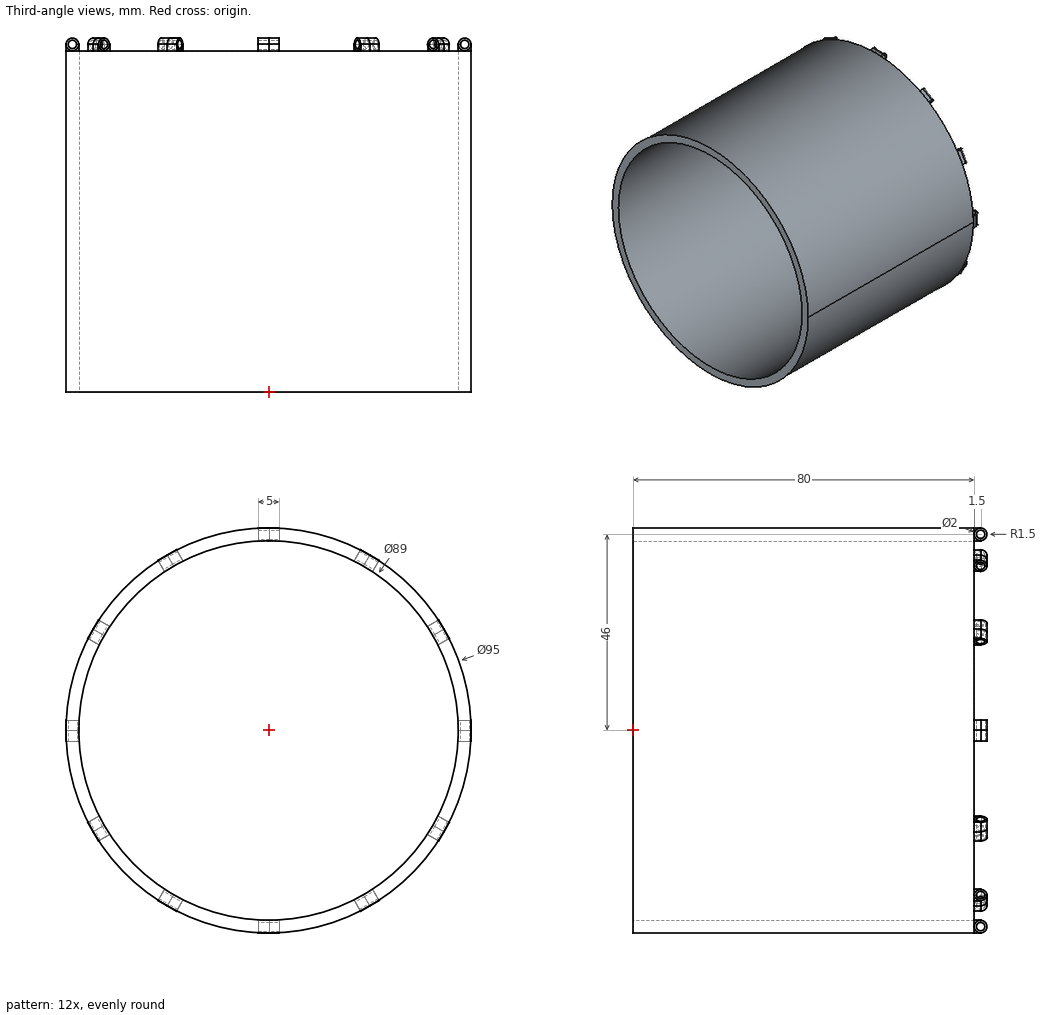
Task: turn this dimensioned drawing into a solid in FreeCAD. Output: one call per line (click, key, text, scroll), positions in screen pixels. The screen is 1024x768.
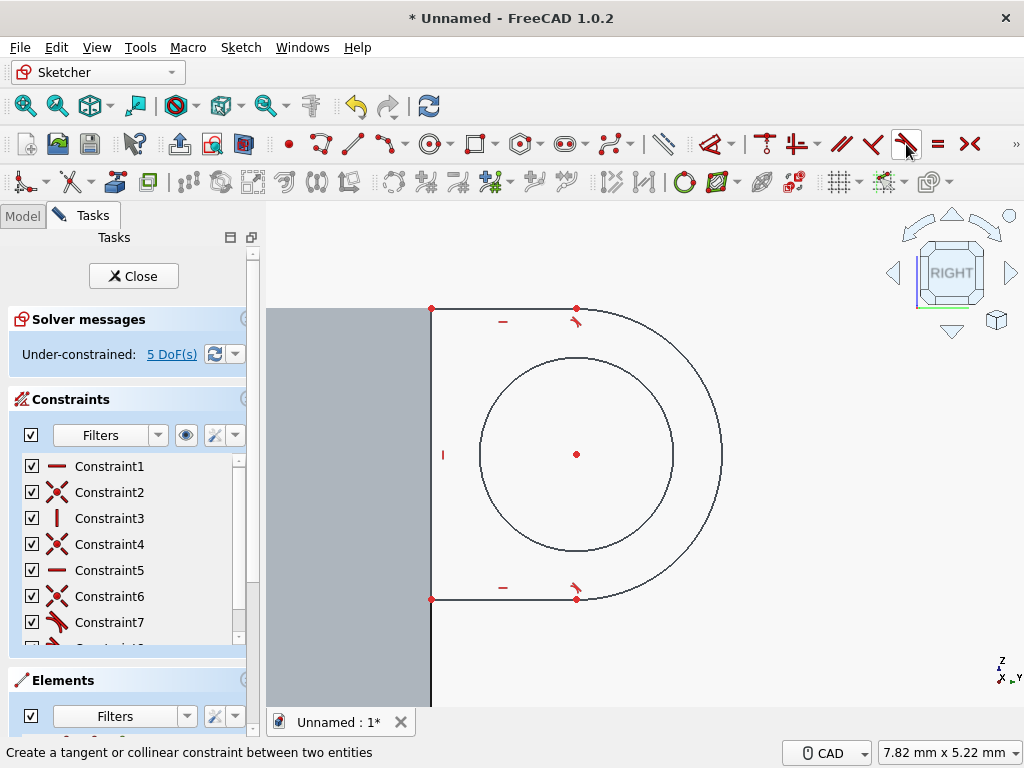
click(710, 144)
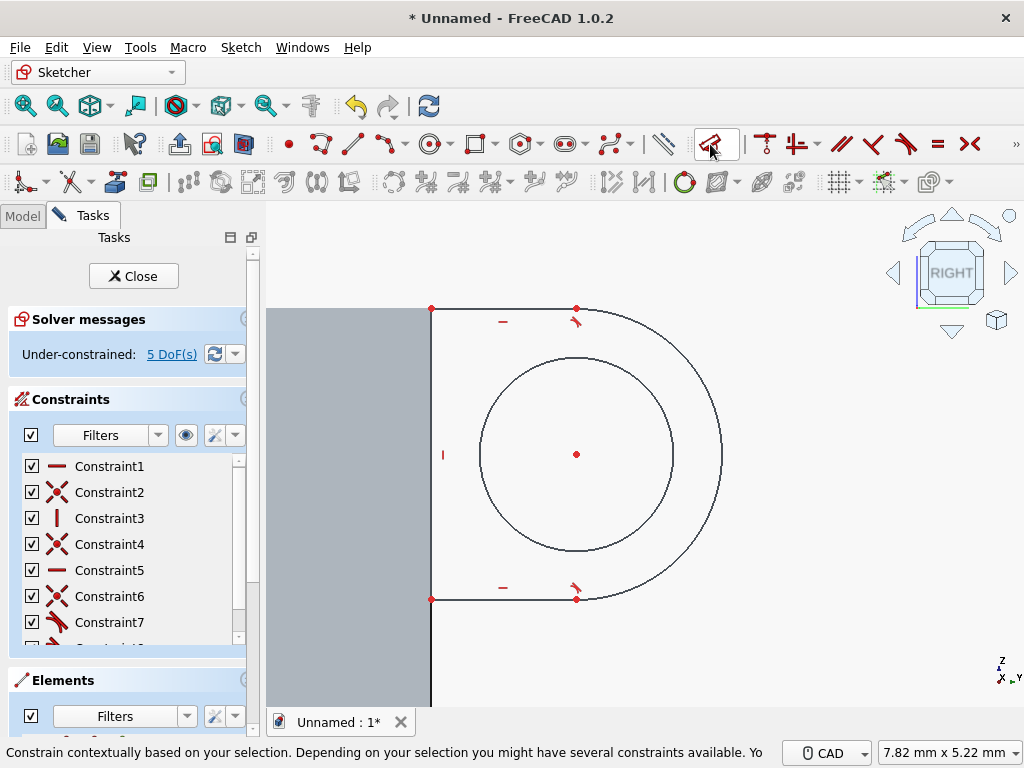
click(694, 540)
click(720, 559)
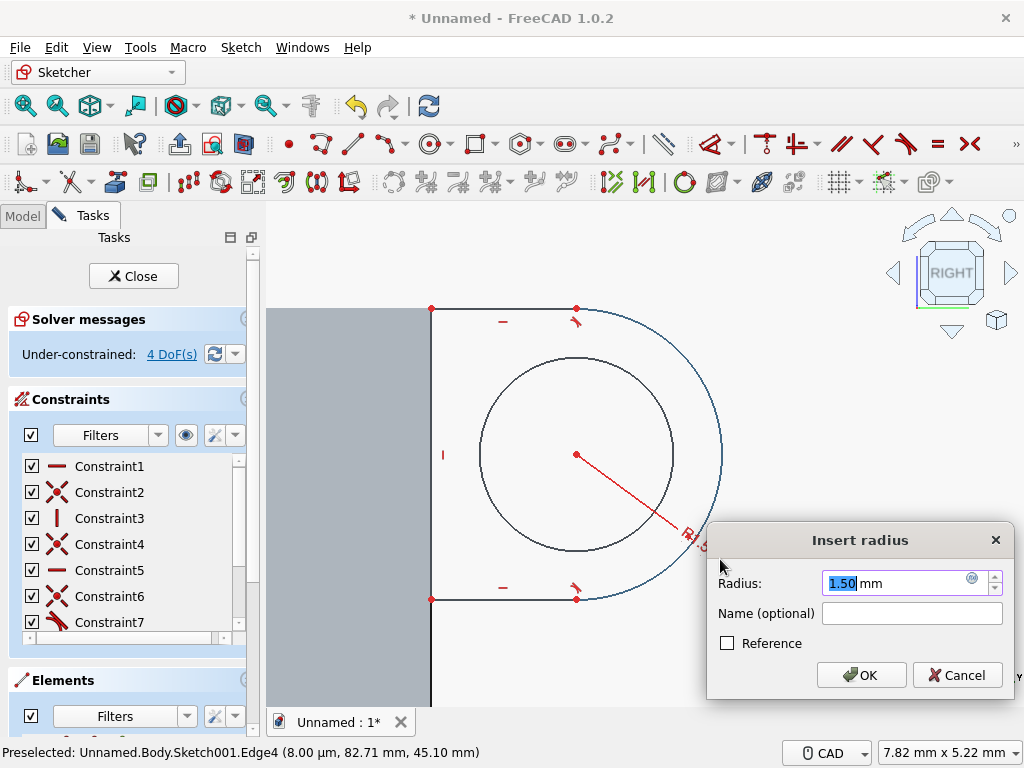
text(1.5)
key(Return)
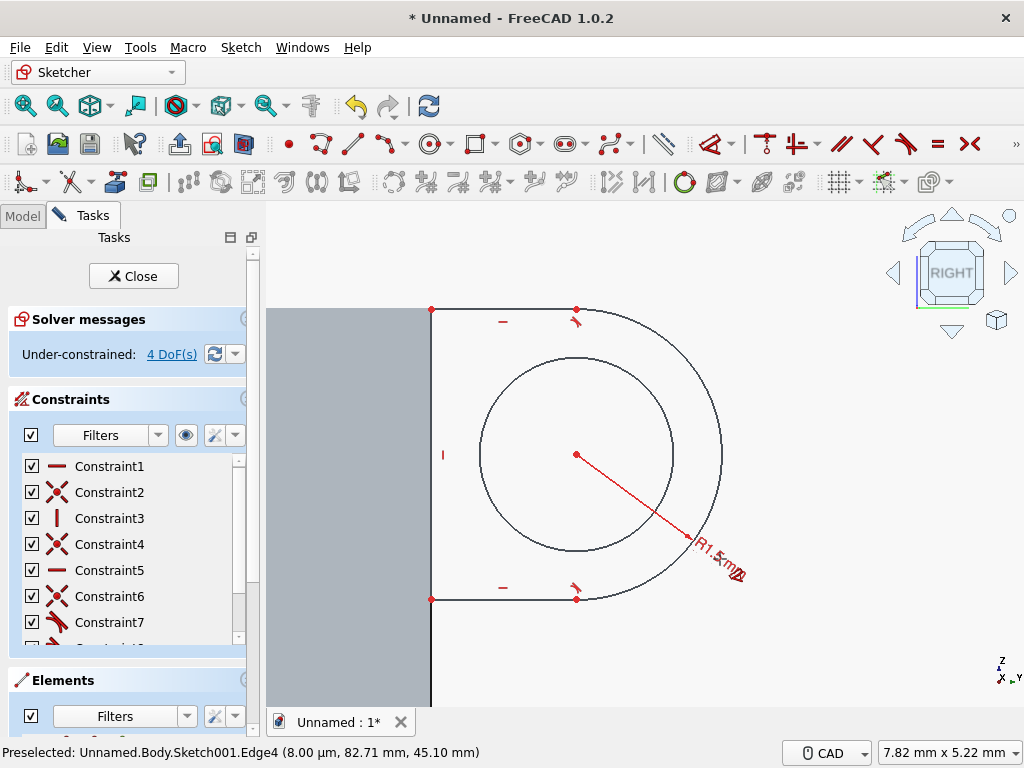
click(645, 386)
click(668, 363)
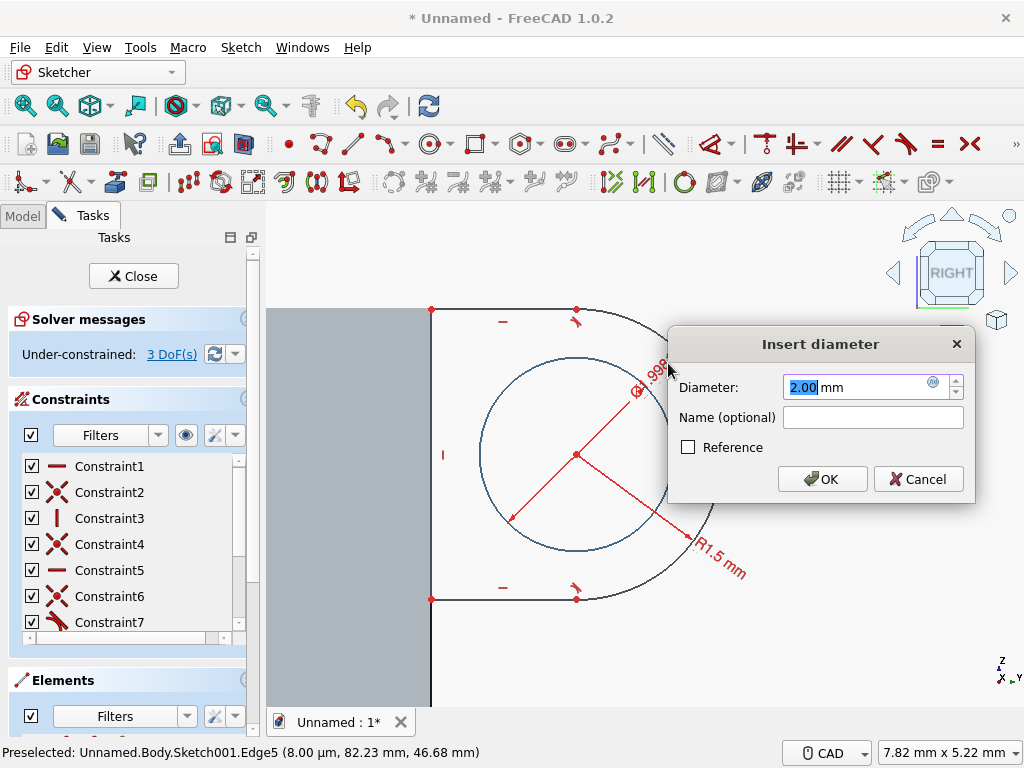
text(2)
key(Return)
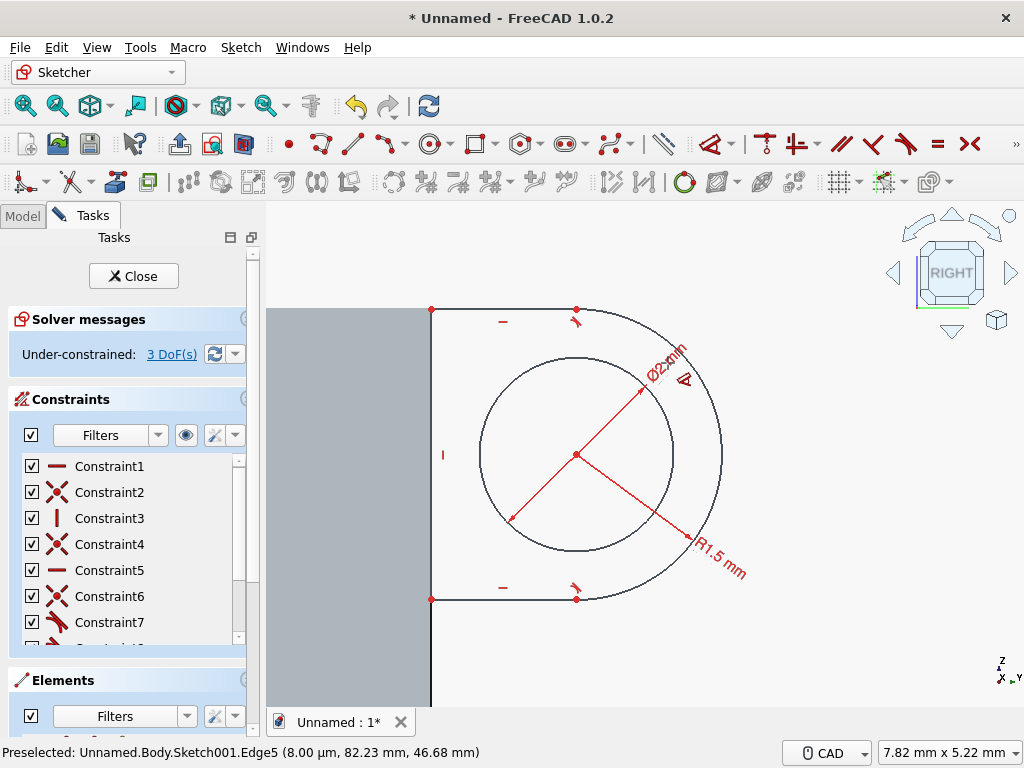
click(576, 455)
click(610, 567)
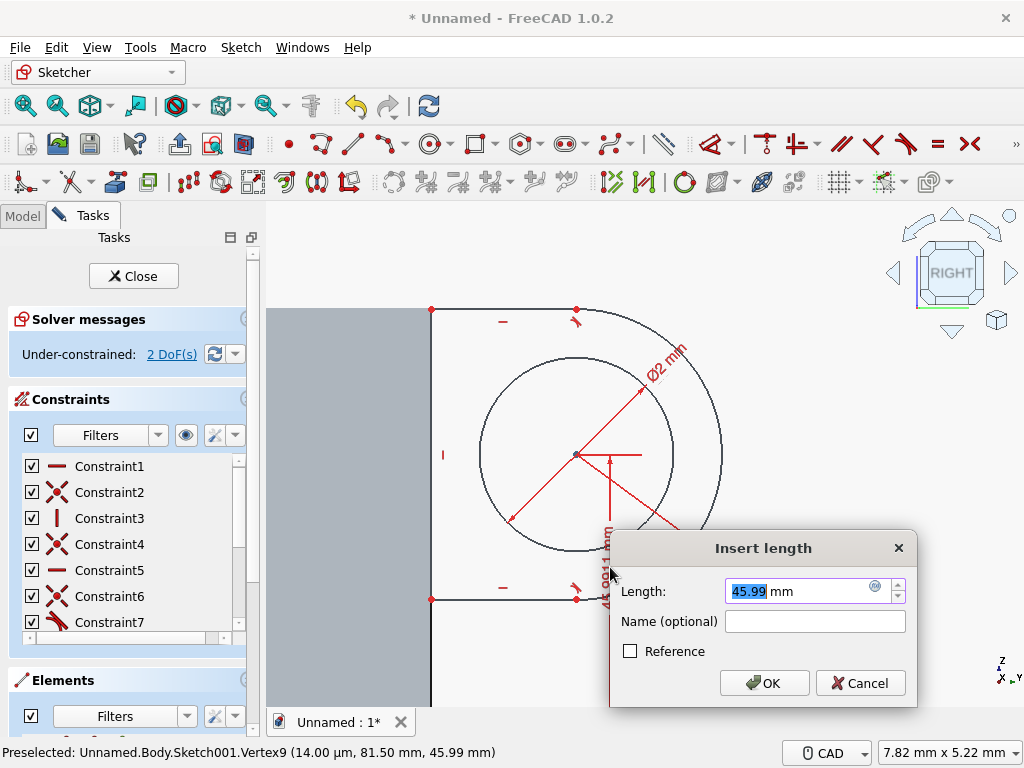
text(46)
key(Return)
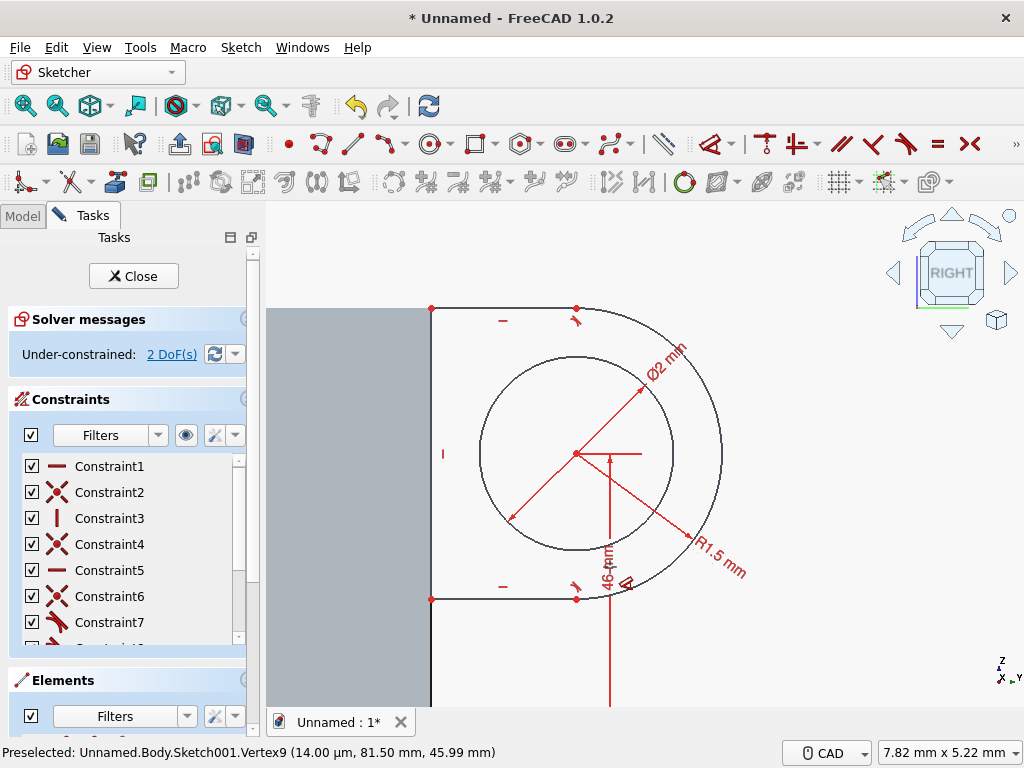
click(533, 308)
click(504, 274)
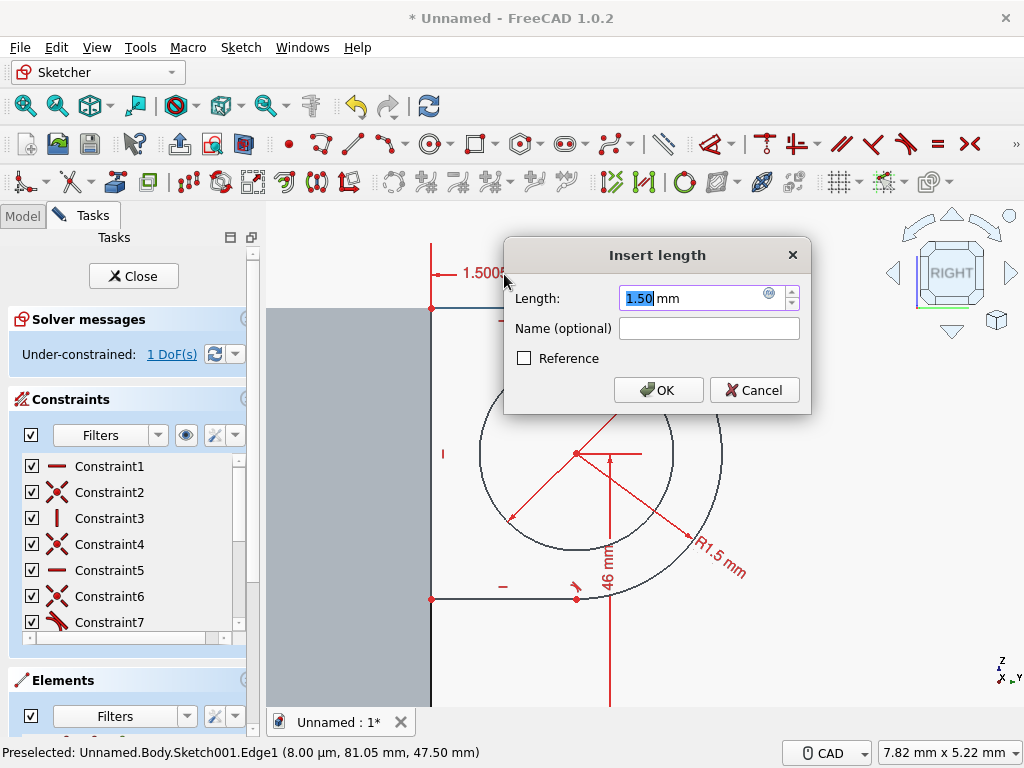
text(1.5)
key(Return)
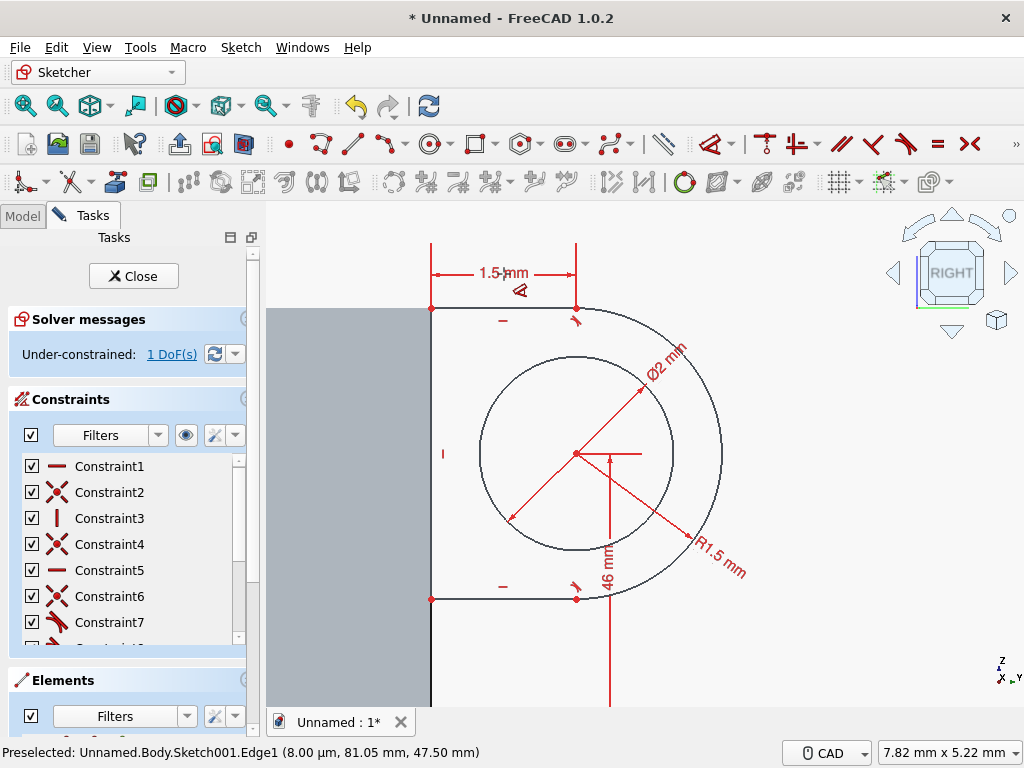
click(431, 308)
click(363, 274)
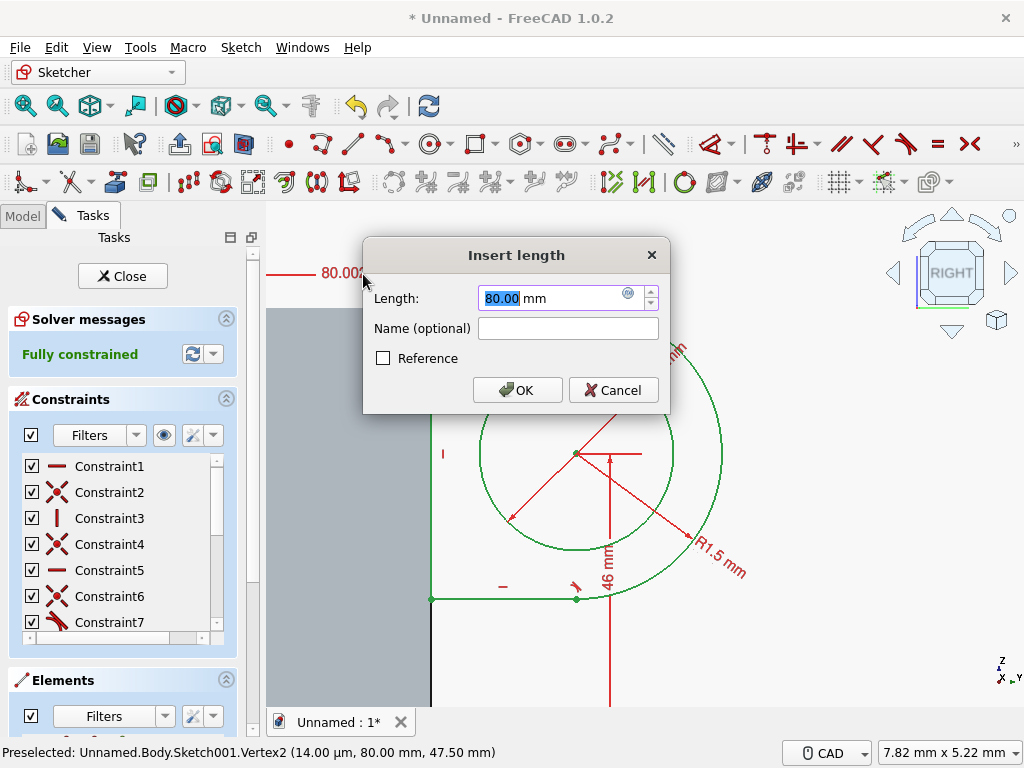
text(80)
key(Return)
key(Escape)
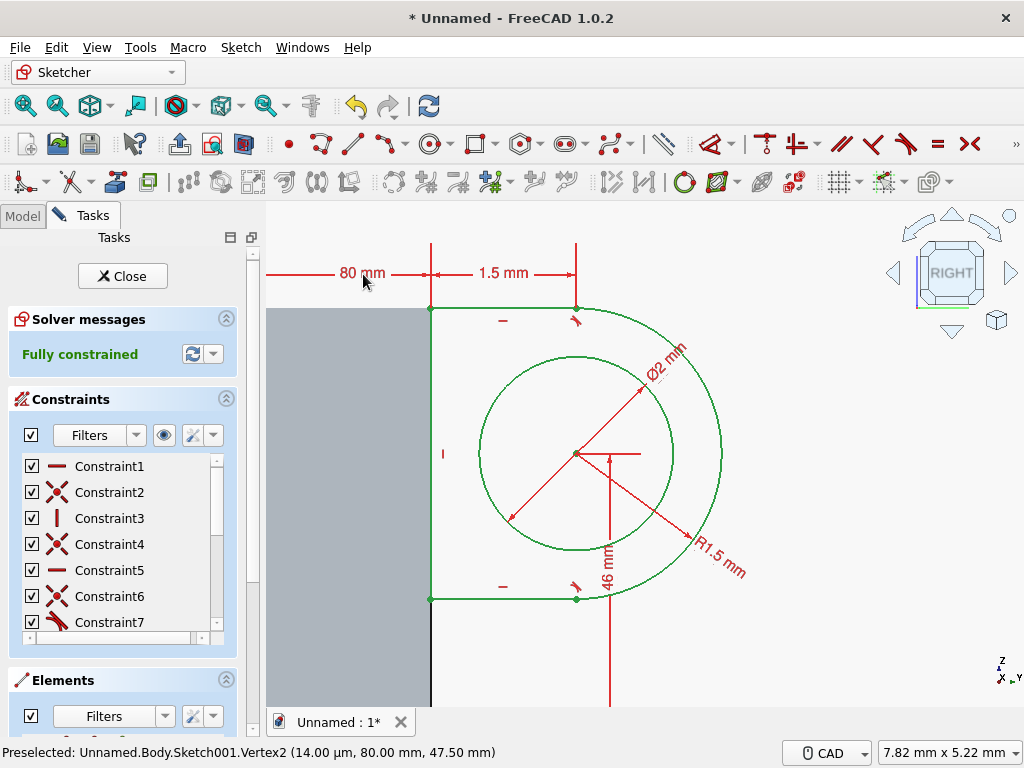
click(123, 276)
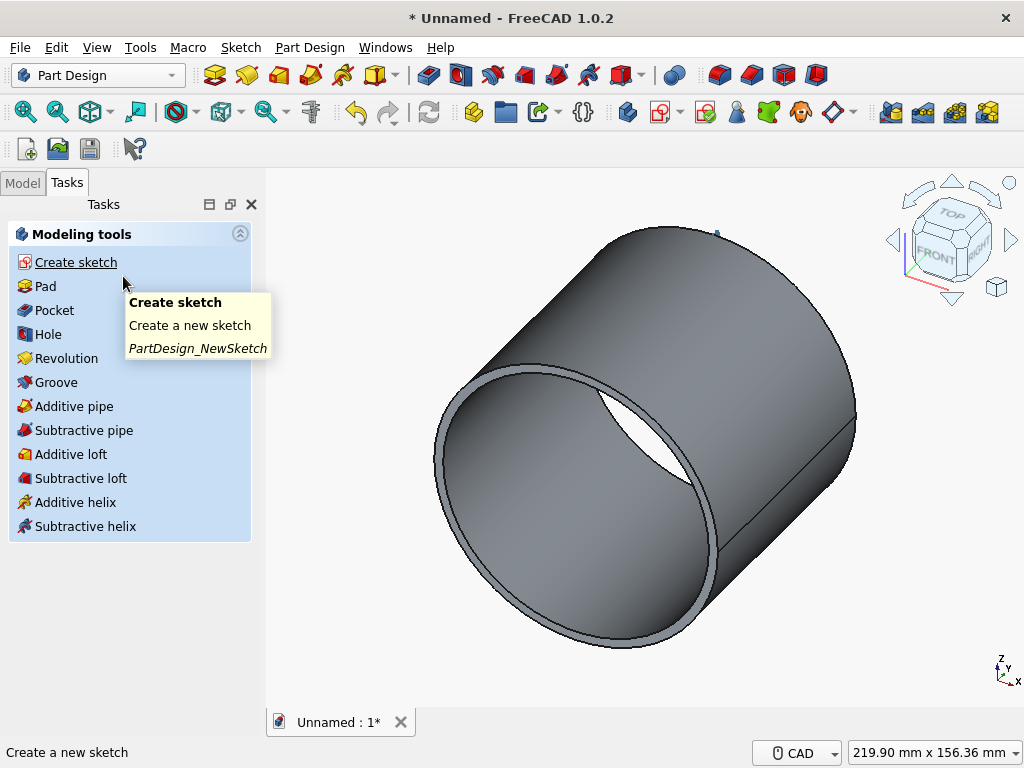
click(216, 76)